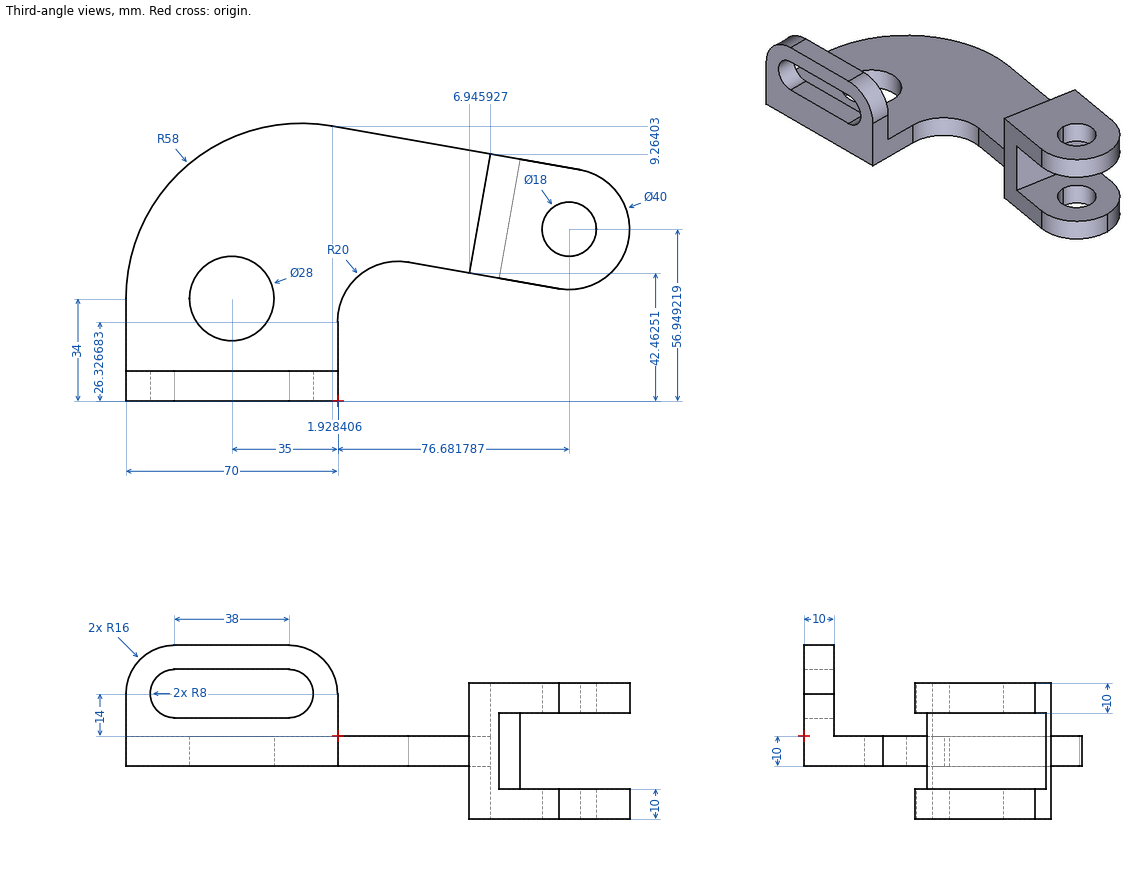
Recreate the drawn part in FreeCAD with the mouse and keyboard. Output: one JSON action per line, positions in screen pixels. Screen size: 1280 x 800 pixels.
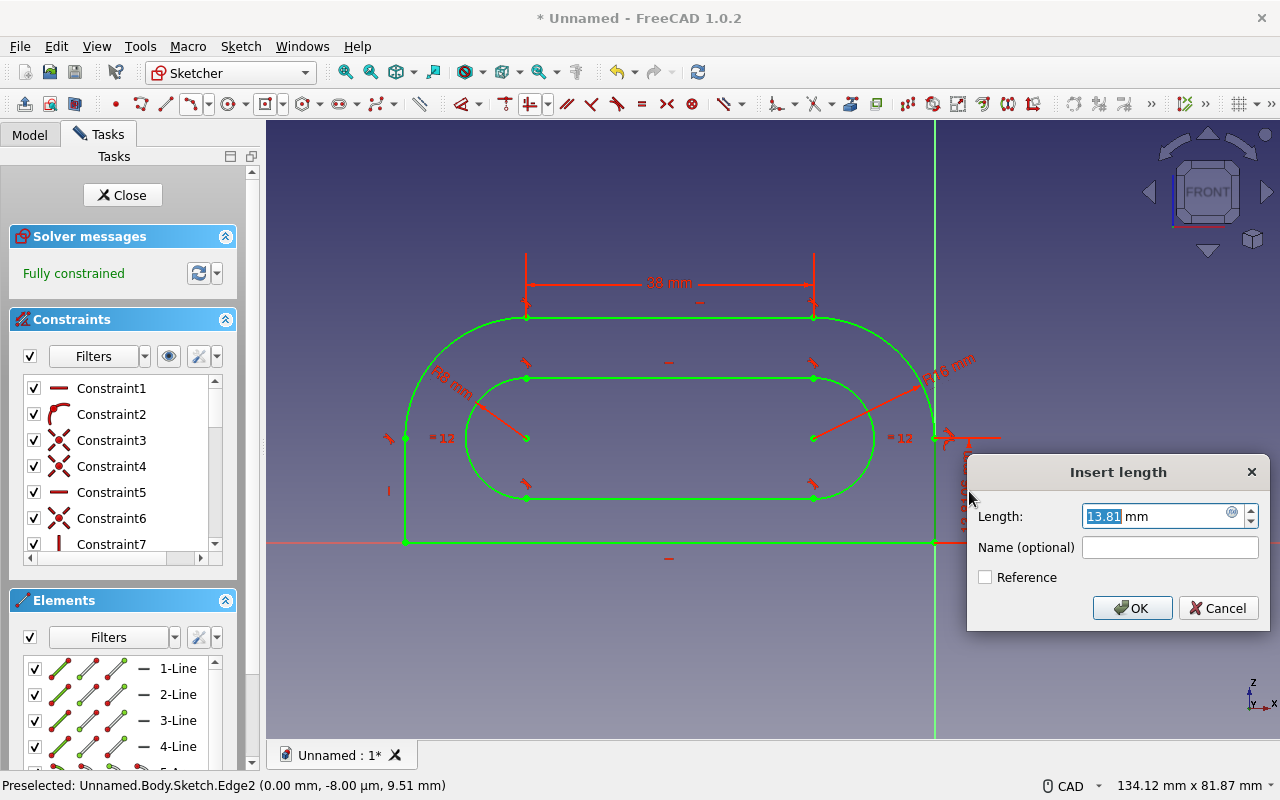
{"action": "type", "text": "14"}
{"action": "key", "text": "Return"}
{"action": "key", "text": "Escape"}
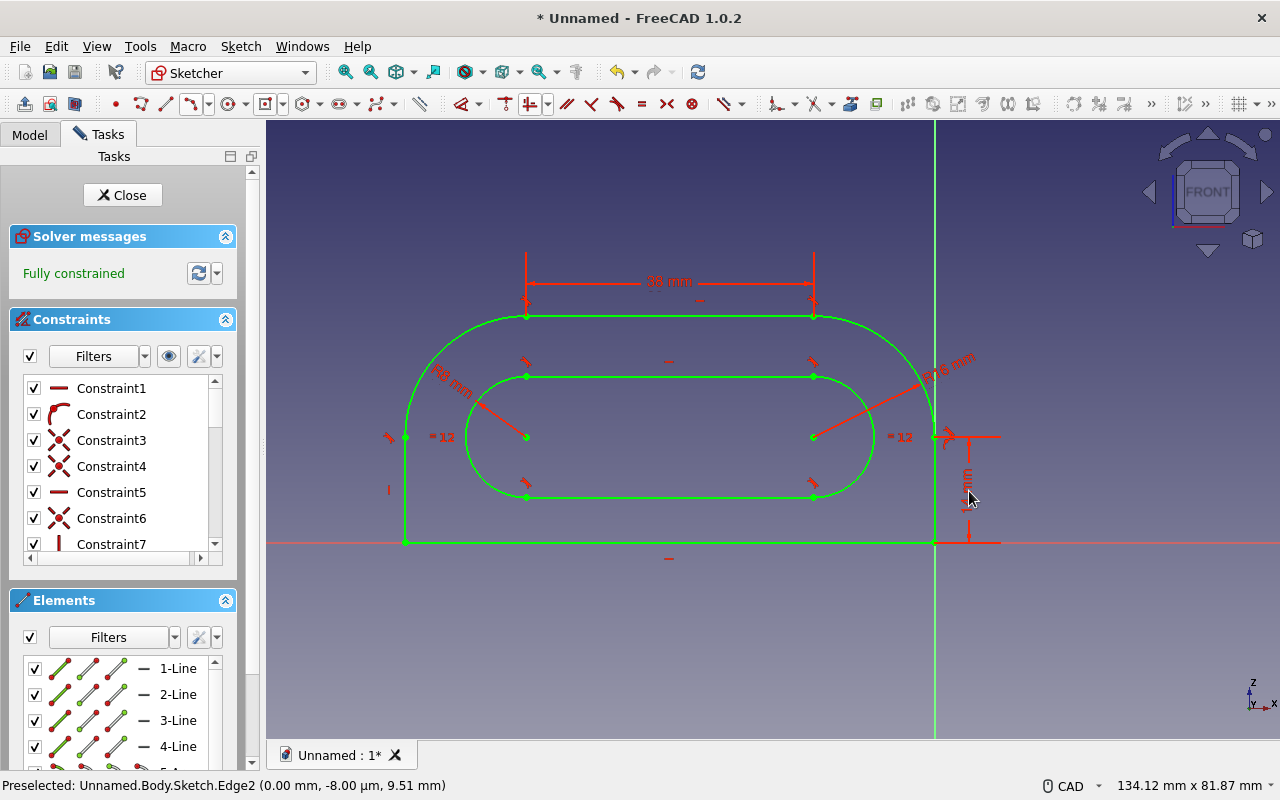
{"action": "left_click", "coordinate": [123, 195]}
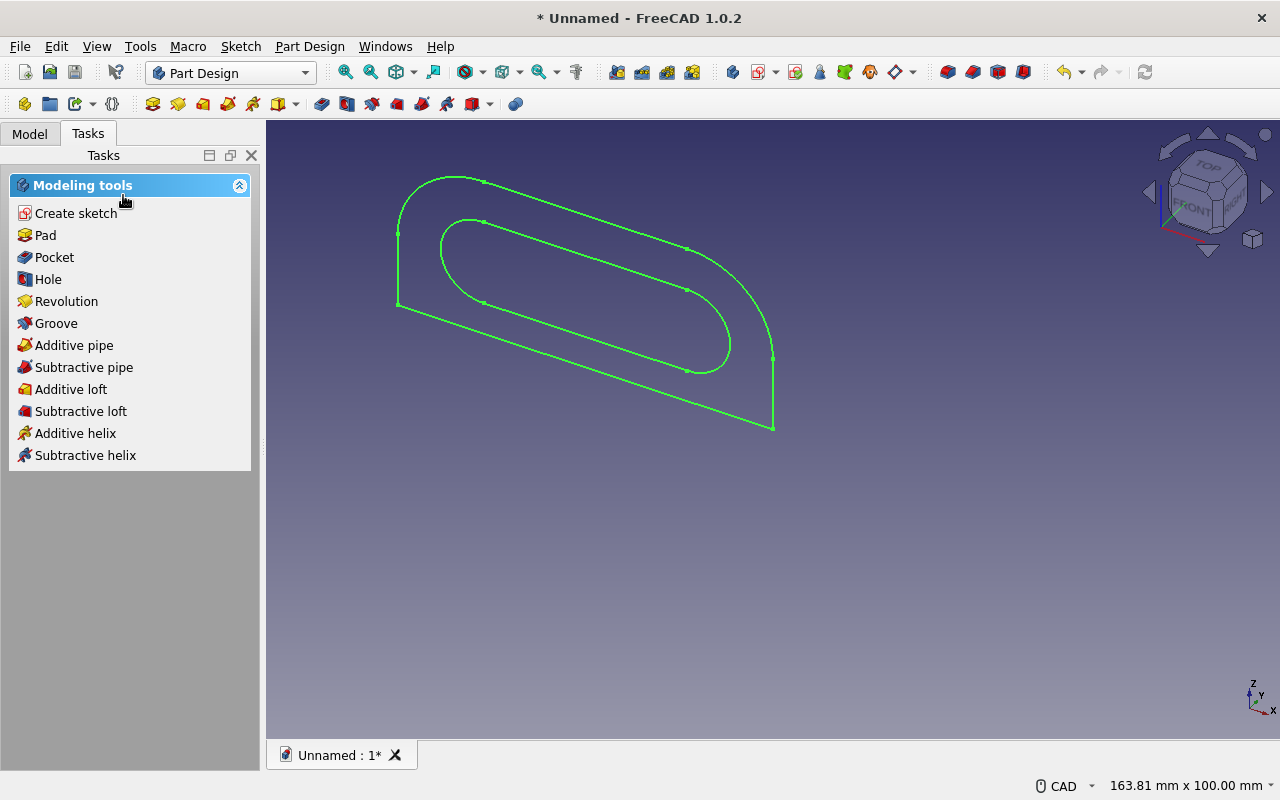
{"action": "left_click", "coordinate": [153, 104]}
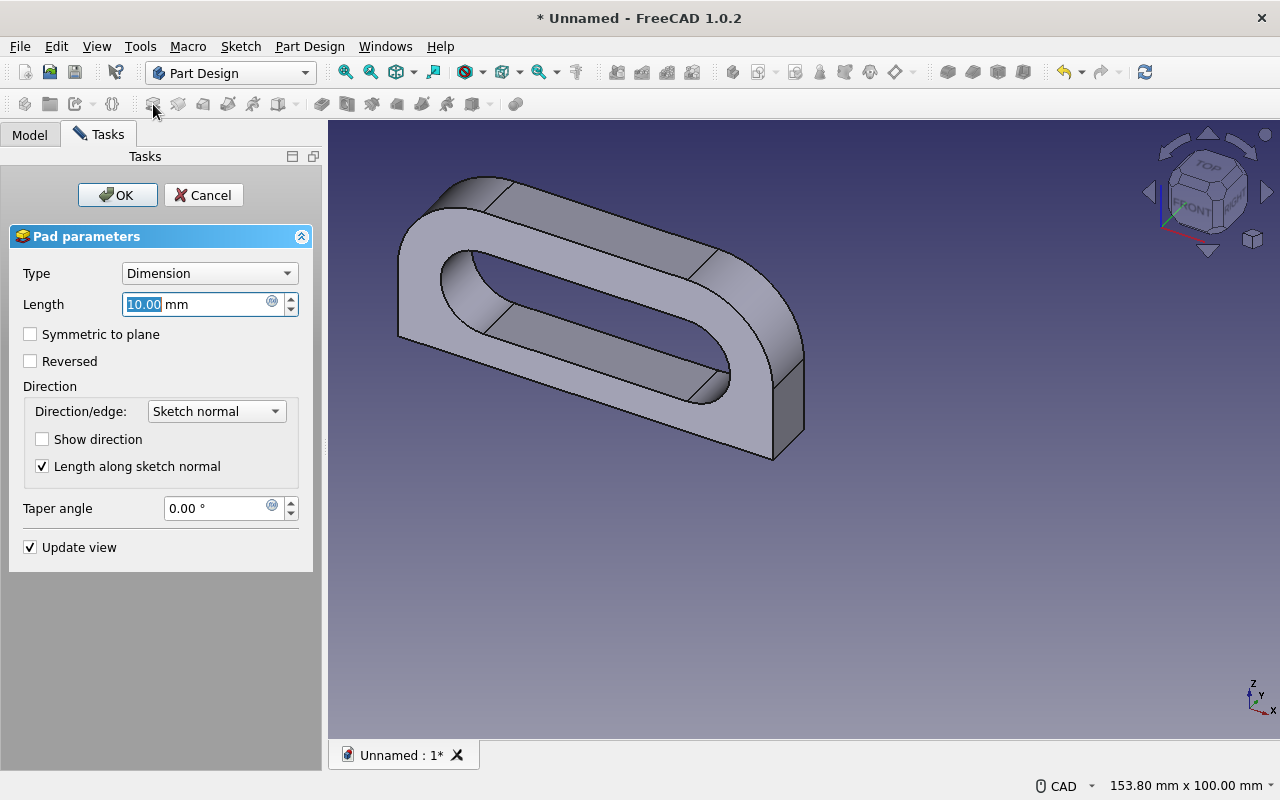
{"action": "type", "text": "10"}
{"action": "key", "text": "Tab"}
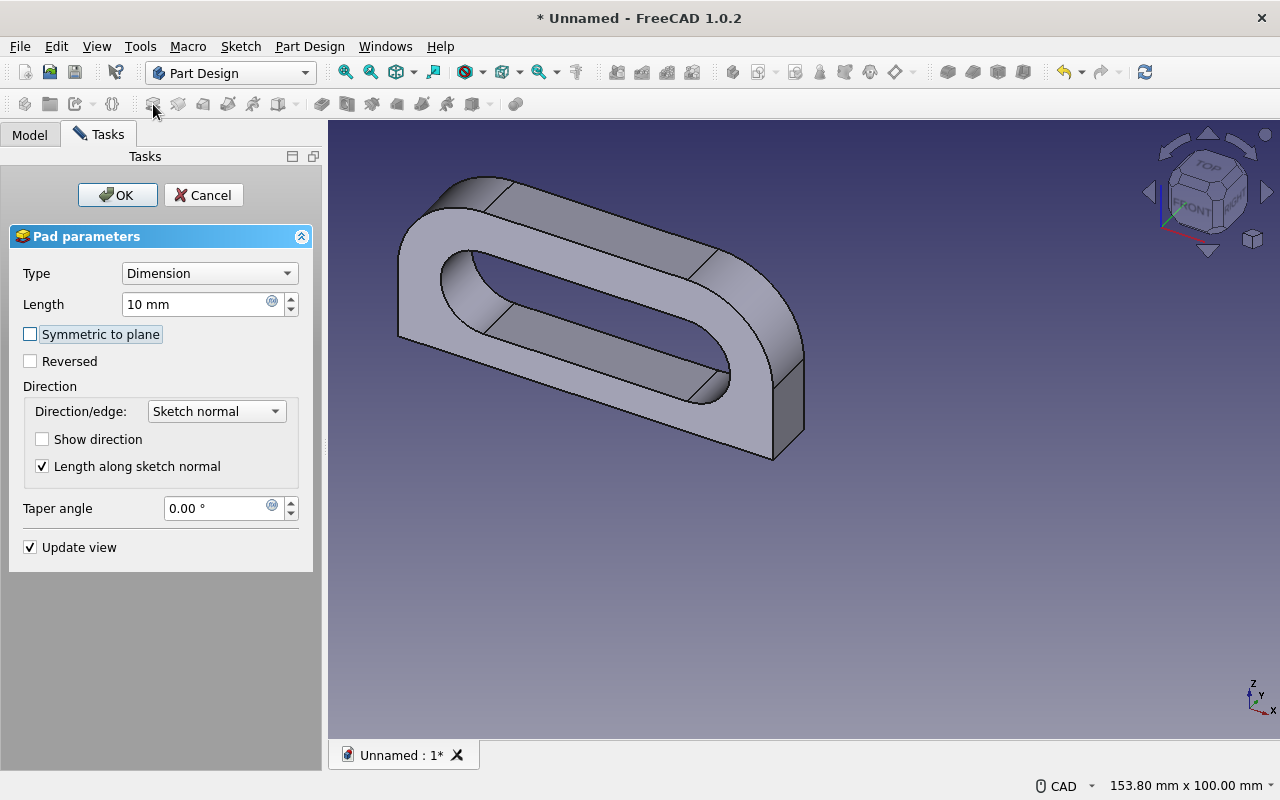
{"action": "left_click", "coordinate": [31, 361]}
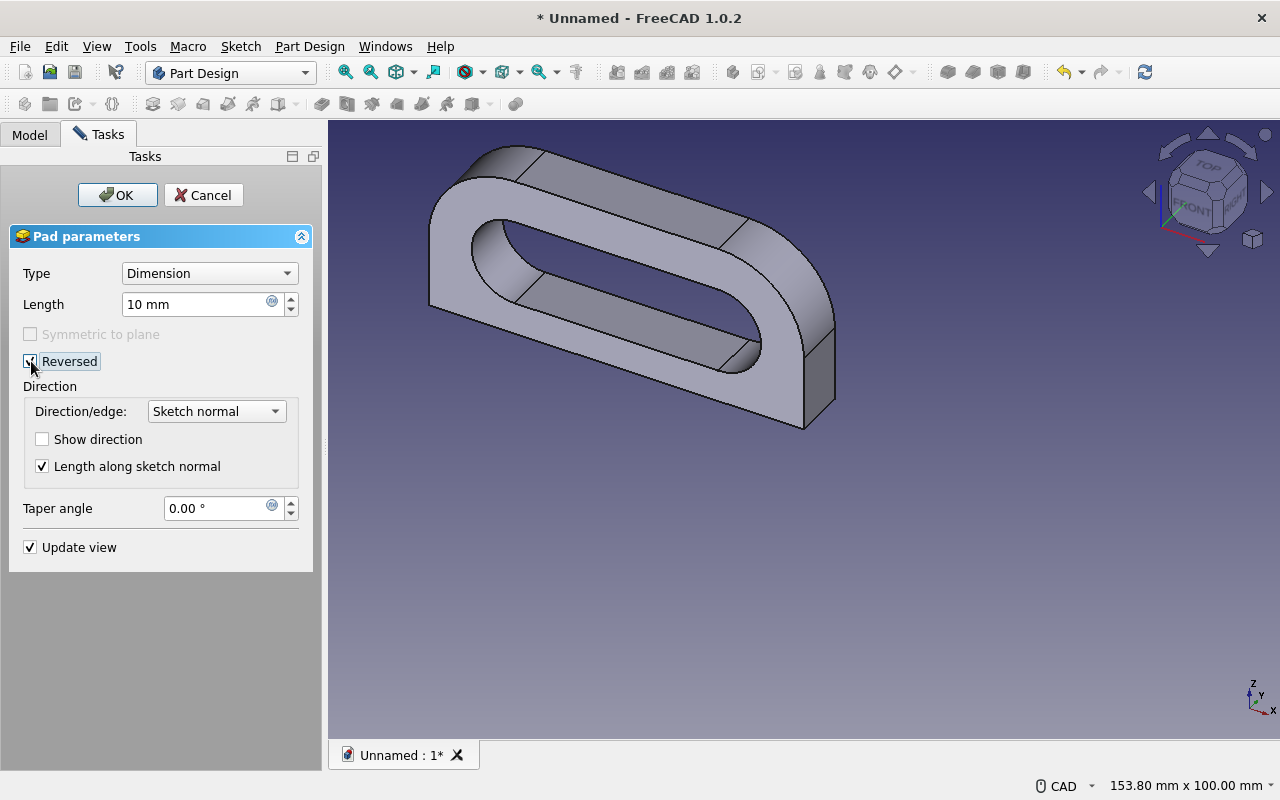
{"action": "left_click", "coordinate": [118, 195]}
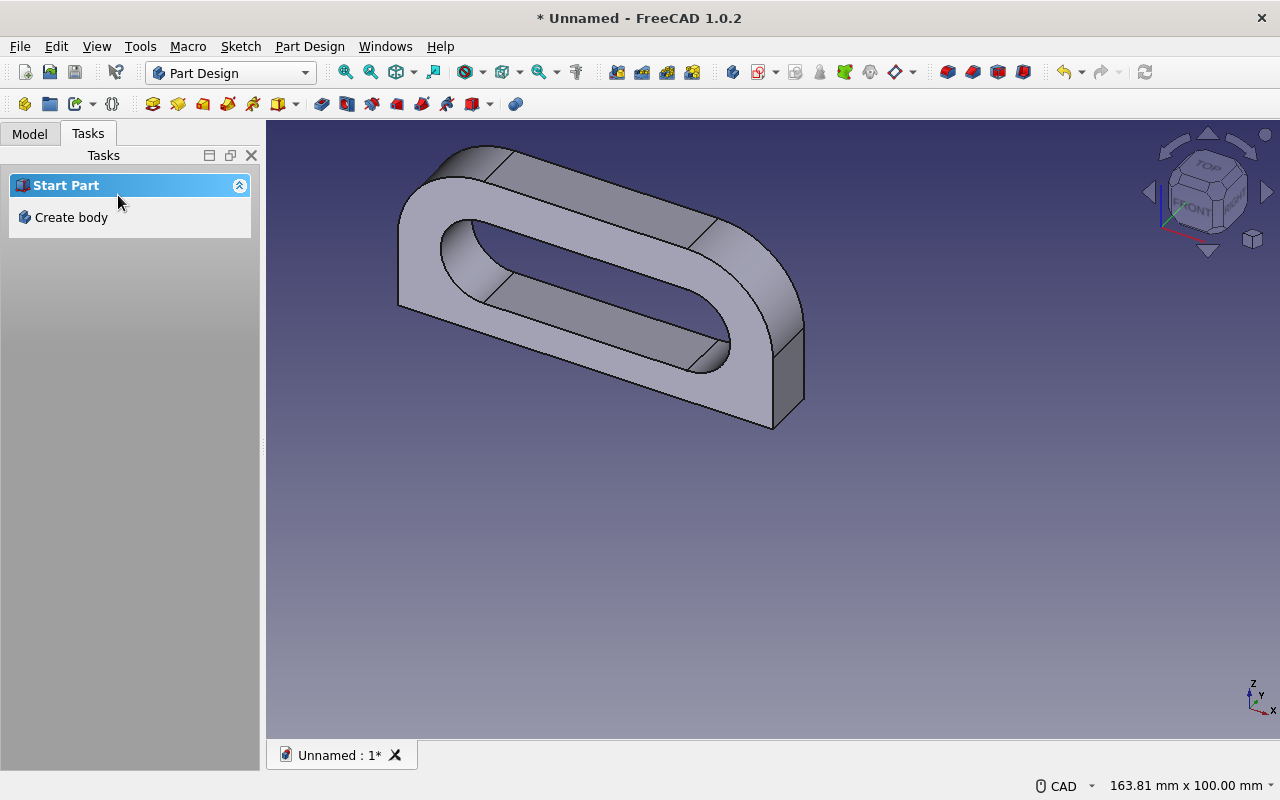
{"action": "key", "text": "5"}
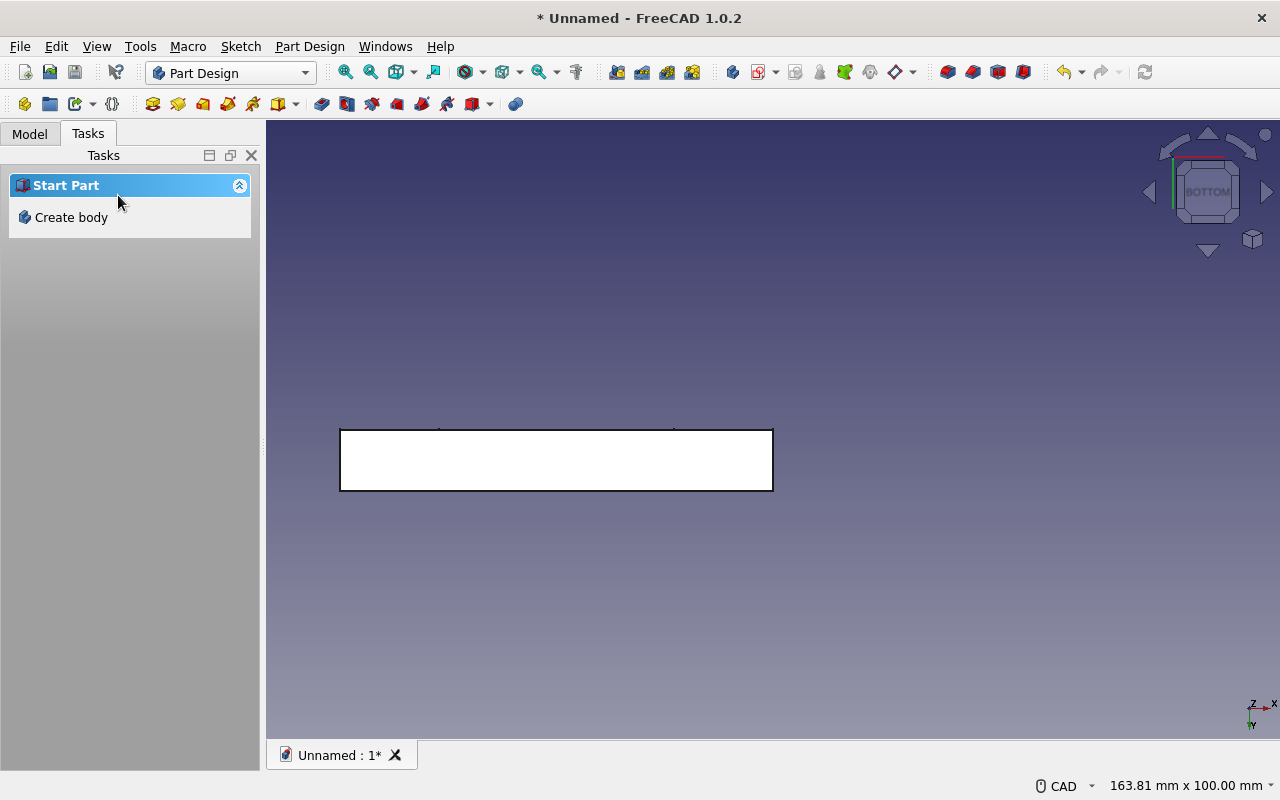
{"action": "left_click", "coordinate": [346, 72]}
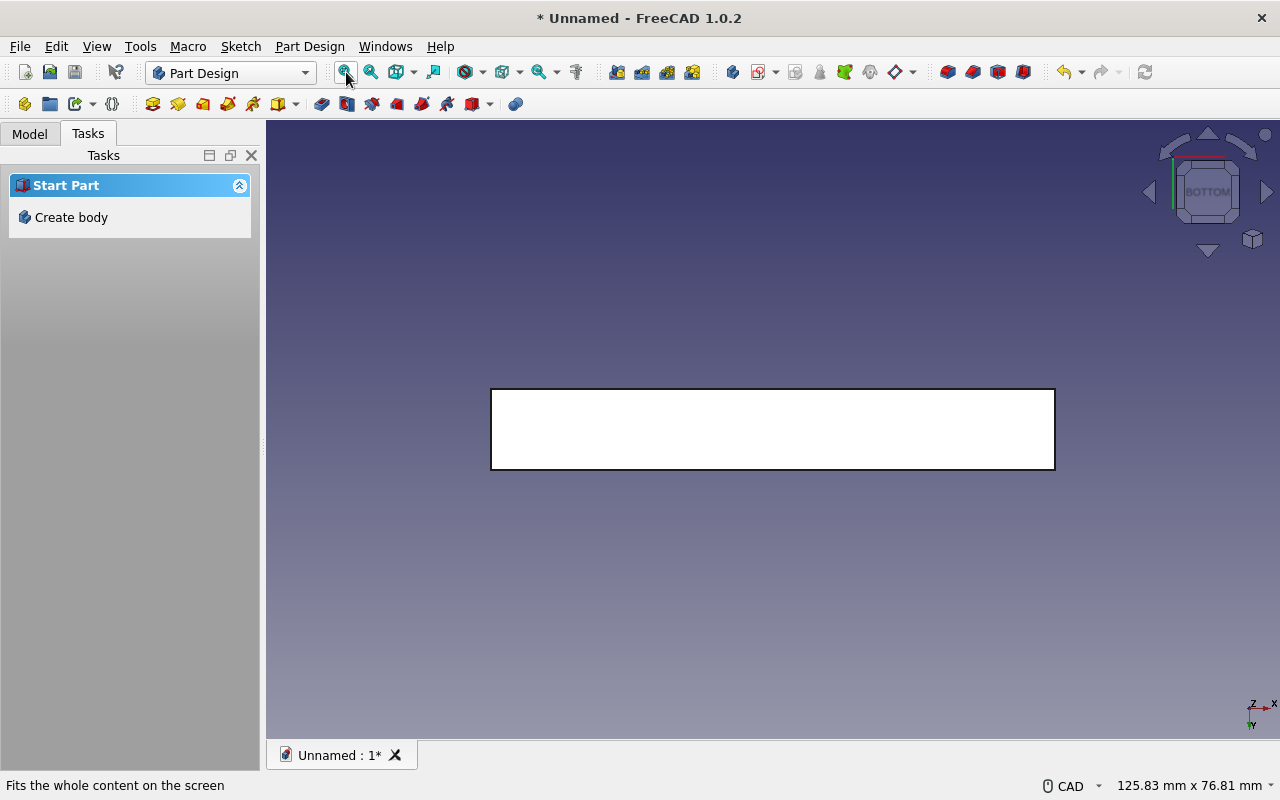
{"action": "left_click", "coordinate": [1015, 429]}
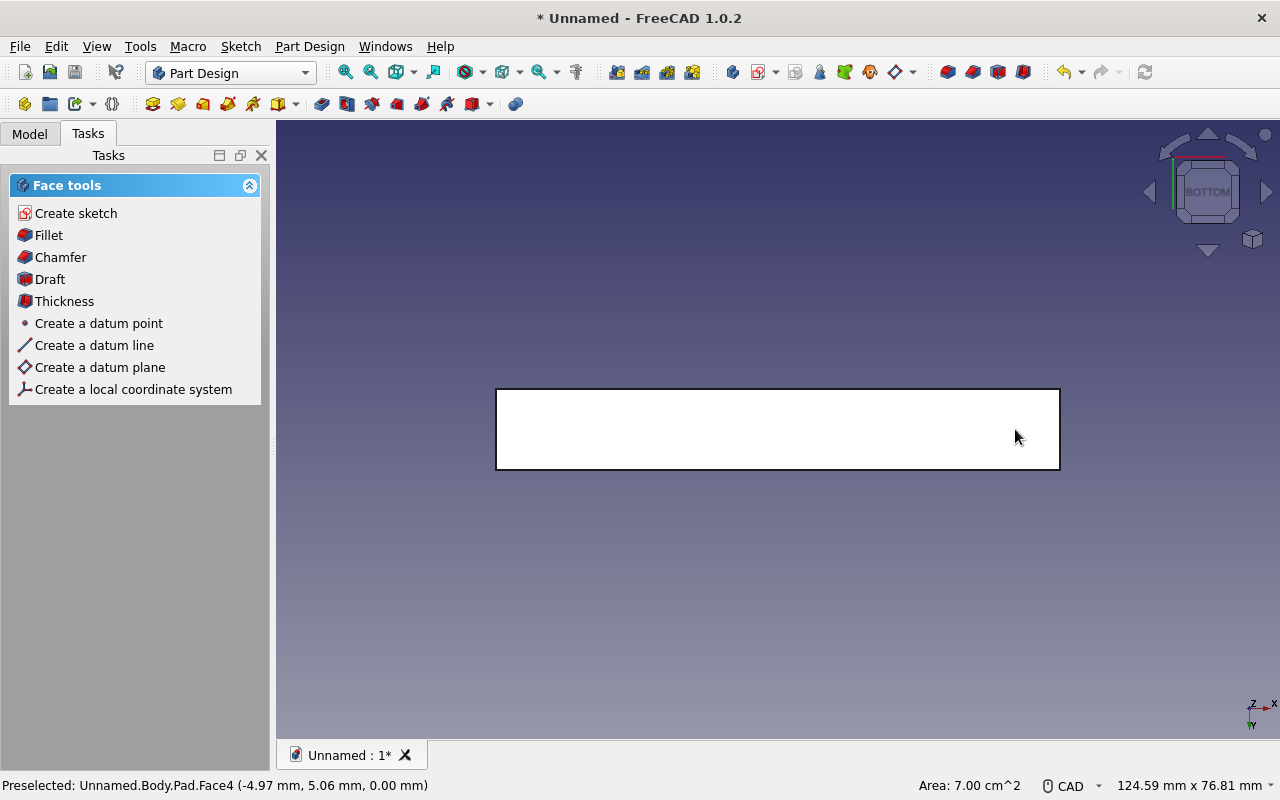
{"action": "left_click", "coordinate": [758, 72]}